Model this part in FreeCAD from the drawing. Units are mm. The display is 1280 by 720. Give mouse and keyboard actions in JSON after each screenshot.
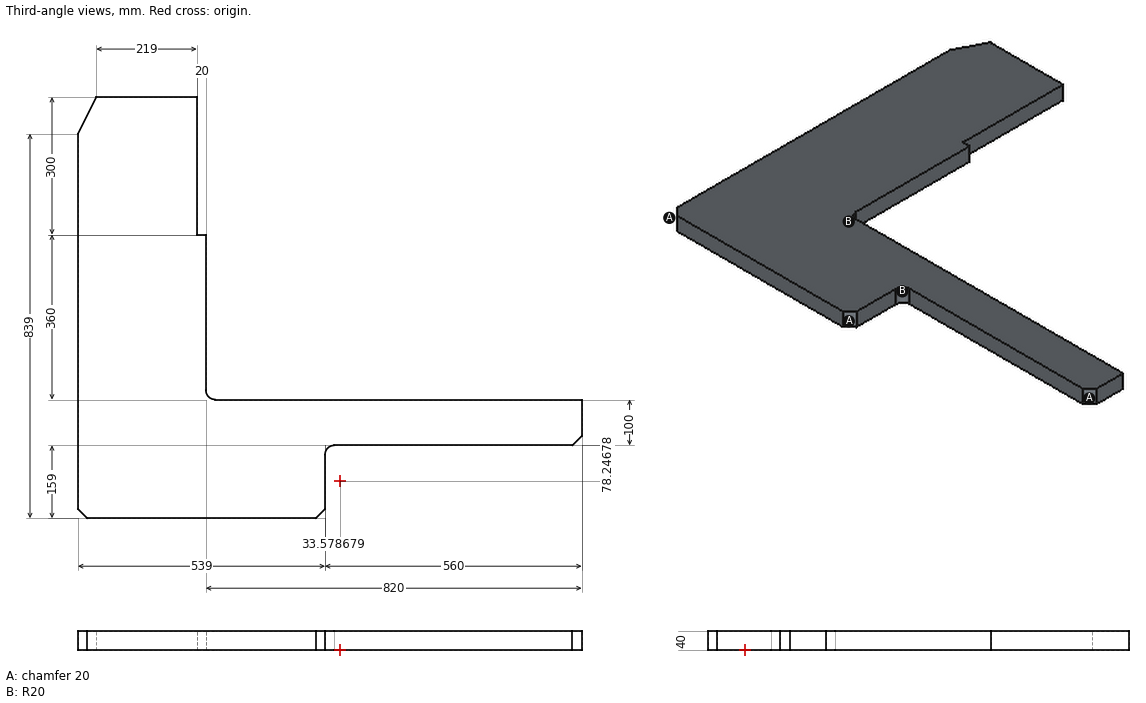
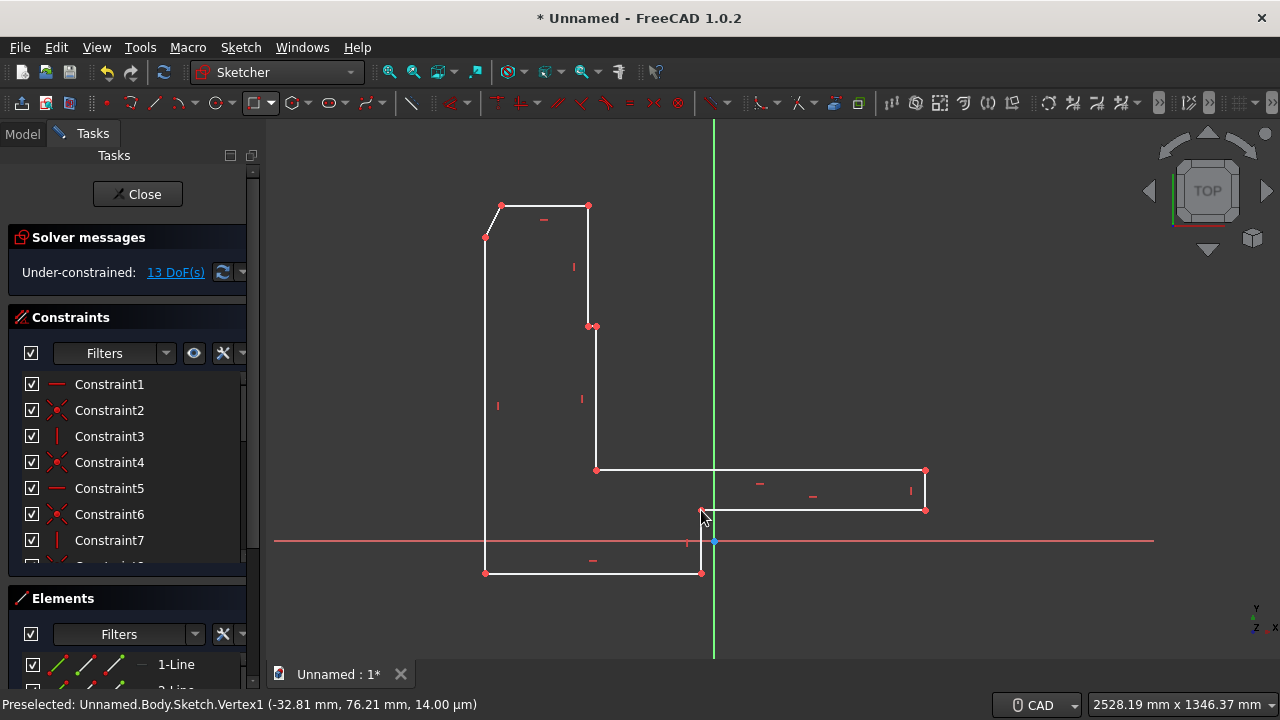
{"action": "scroll", "coordinate": [592, 326], "scroll_direction": "up", "scroll_amount": 7}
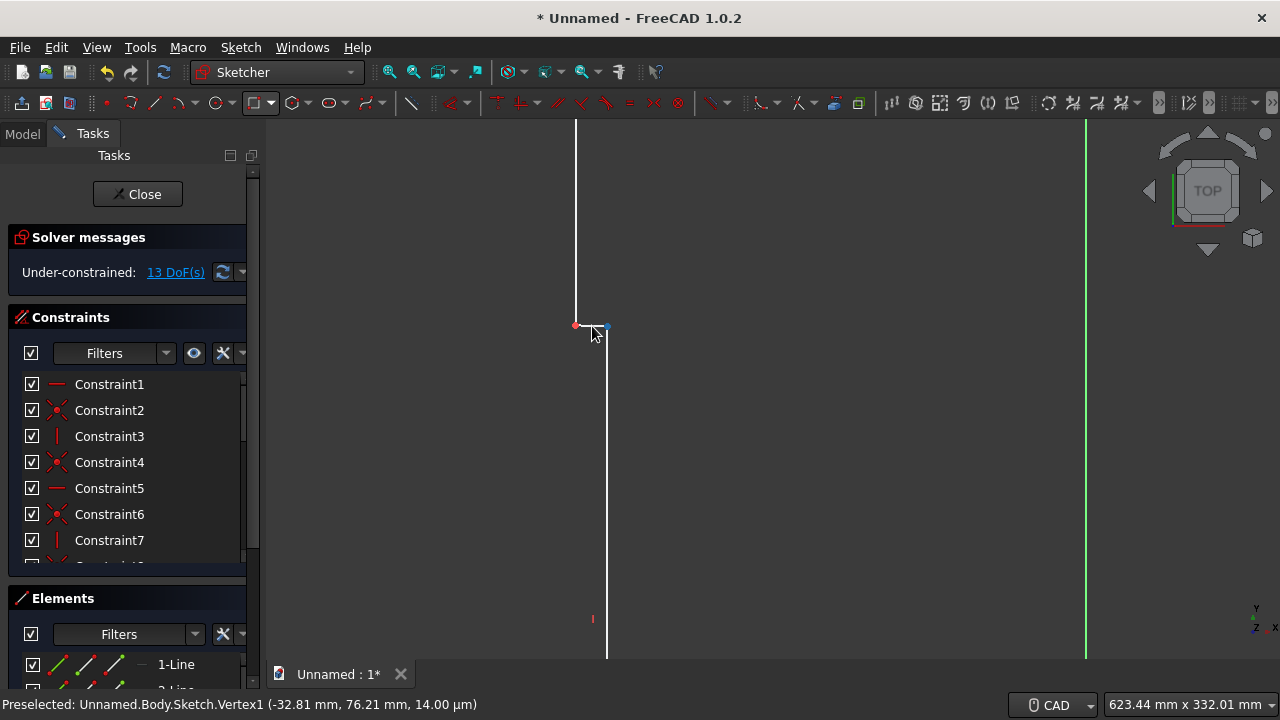
{"action": "left_click", "coordinate": [591, 326]}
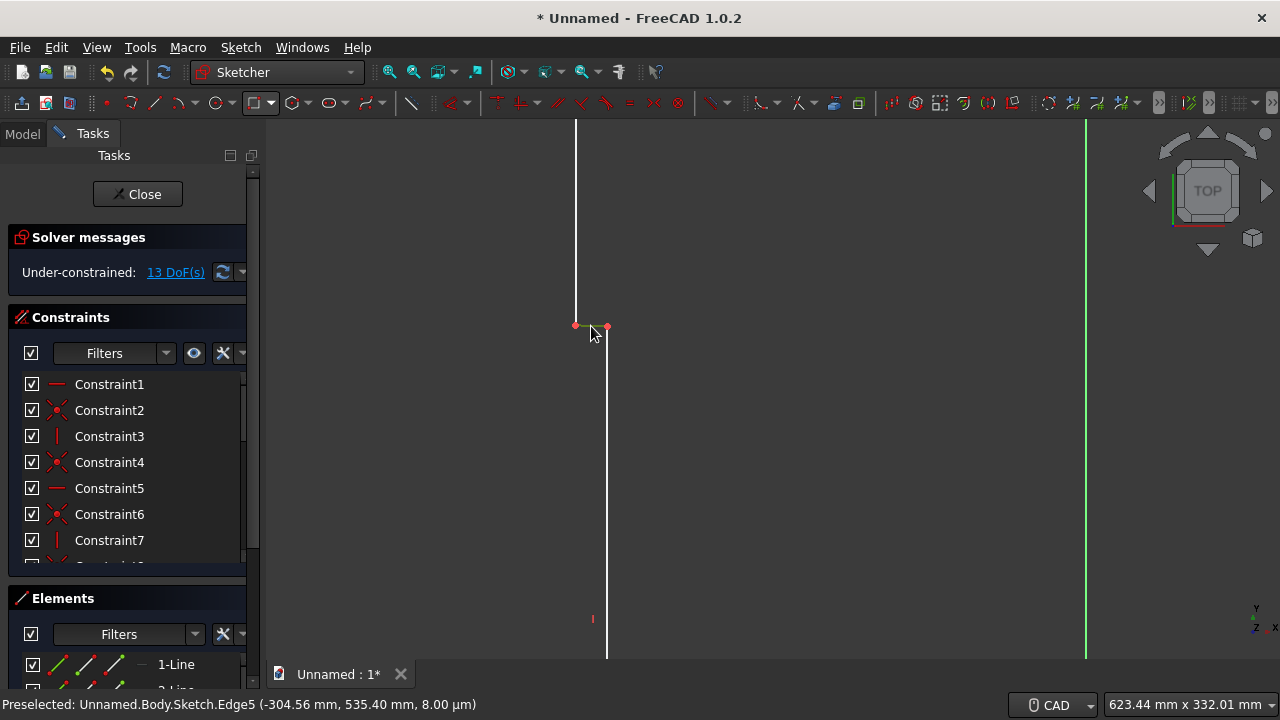
{"action": "key", "text": "h"}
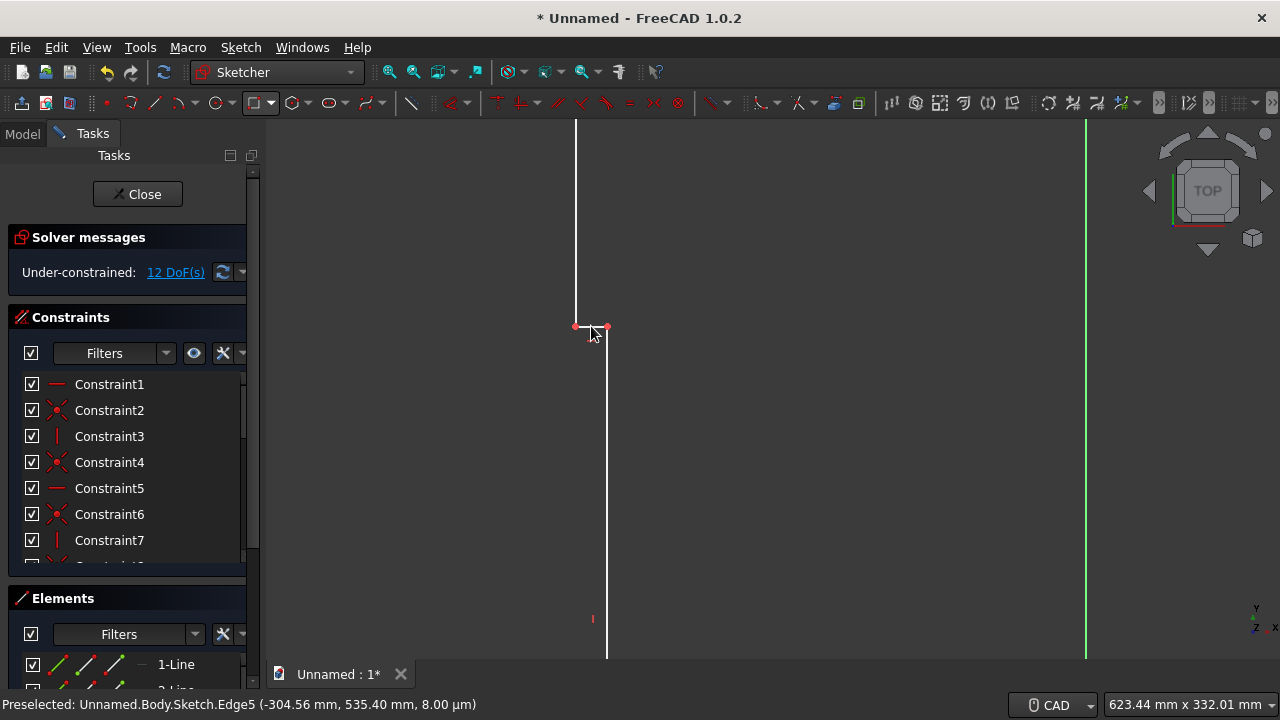
{"action": "key", "text": "d"}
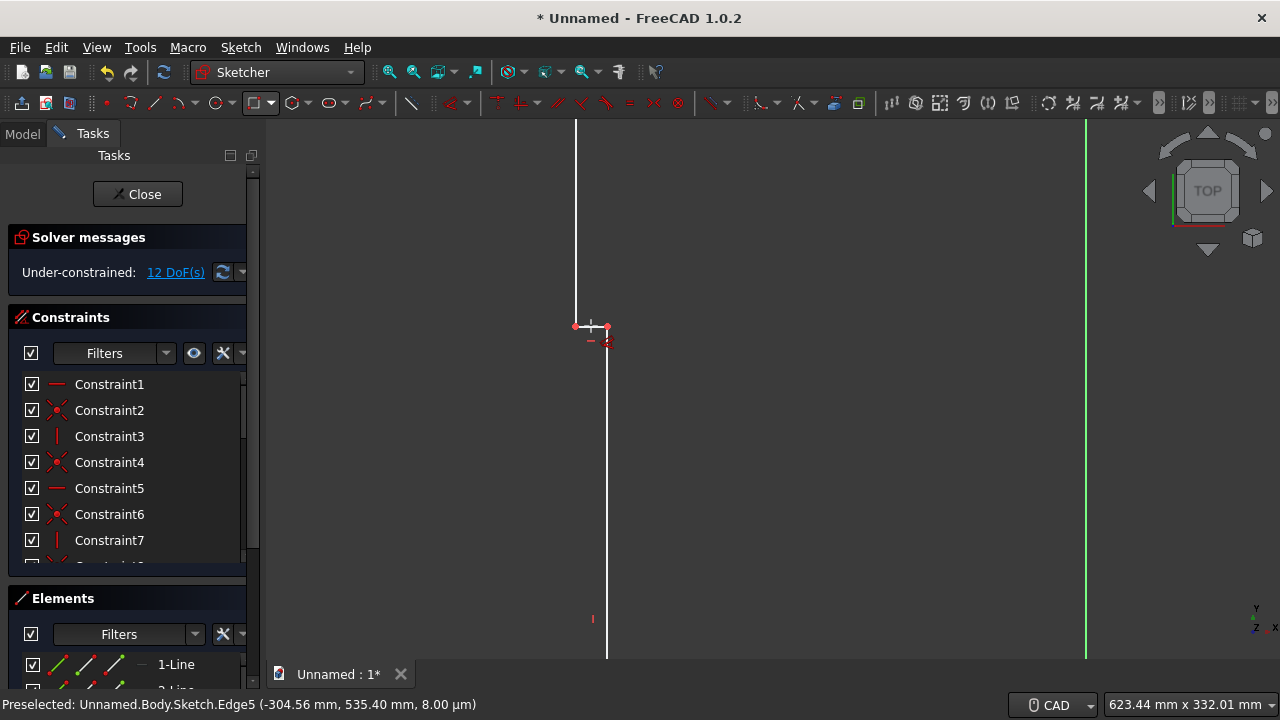
{"action": "scroll", "coordinate": [598, 327], "scroll_direction": "up", "scroll_amount": 2}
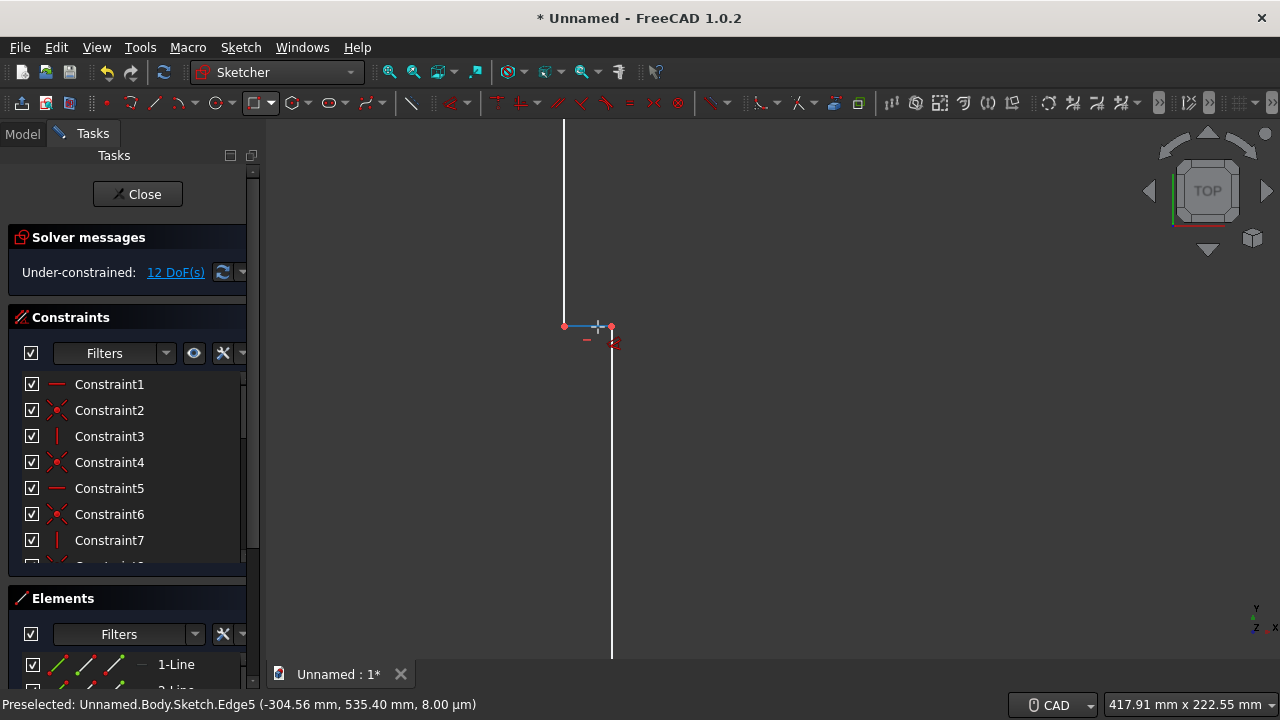
{"action": "left_click", "coordinate": [597, 326]}
{"action": "left_click", "coordinate": [588, 292]}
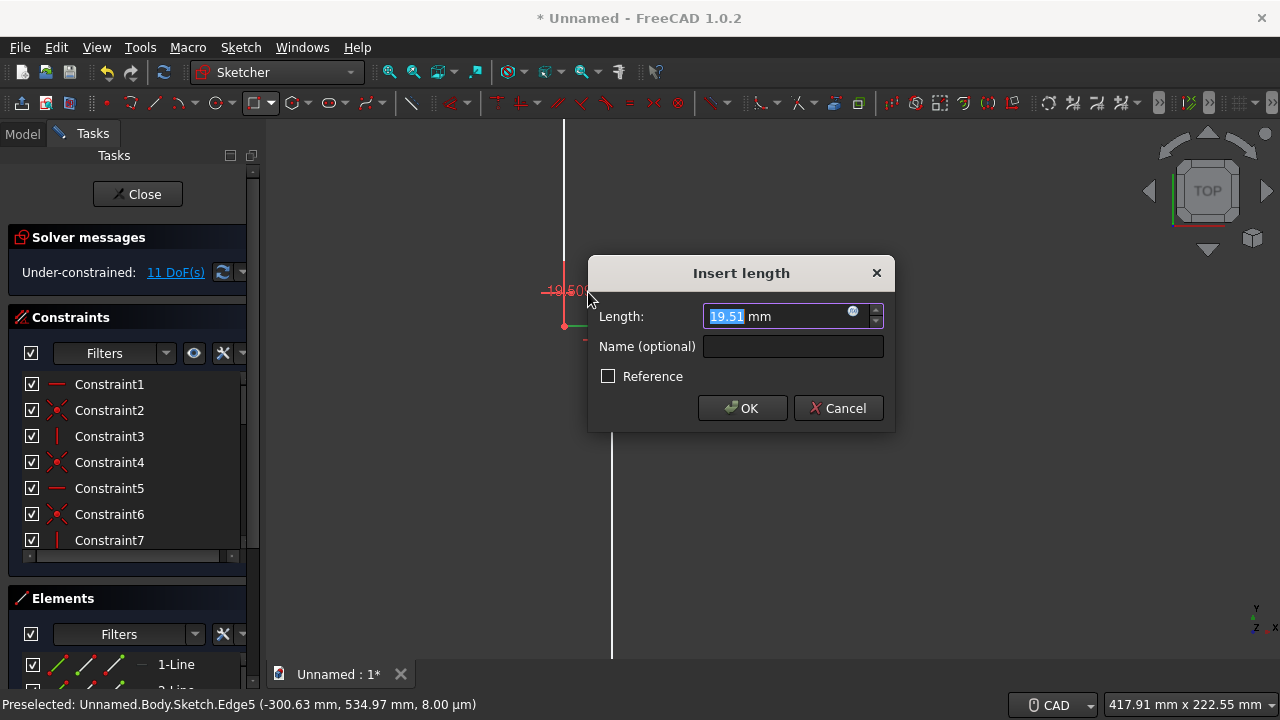
{"action": "type", "text": "20"}
{"action": "key", "text": "Return"}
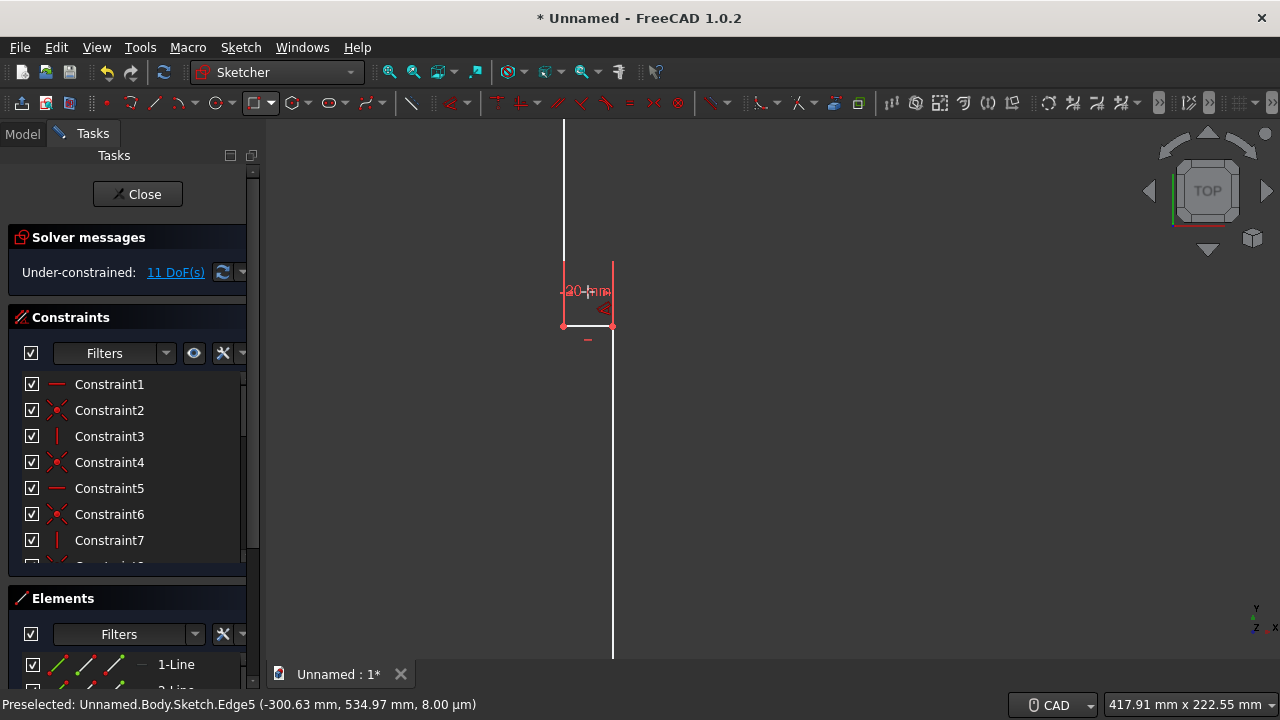
{"action": "scroll", "coordinate": [592, 326], "scroll_direction": "down", "scroll_amount": 9}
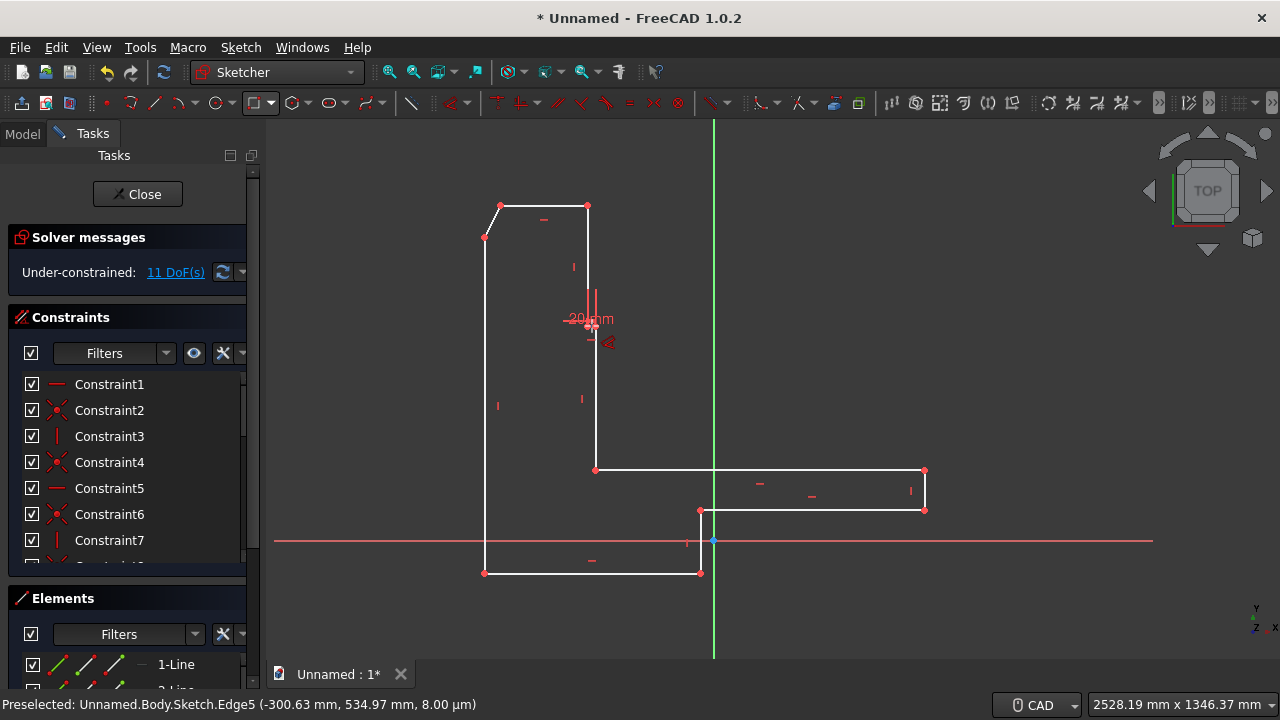
{"action": "left_click", "coordinate": [768, 510]}
{"action": "left_click", "coordinate": [813, 568]}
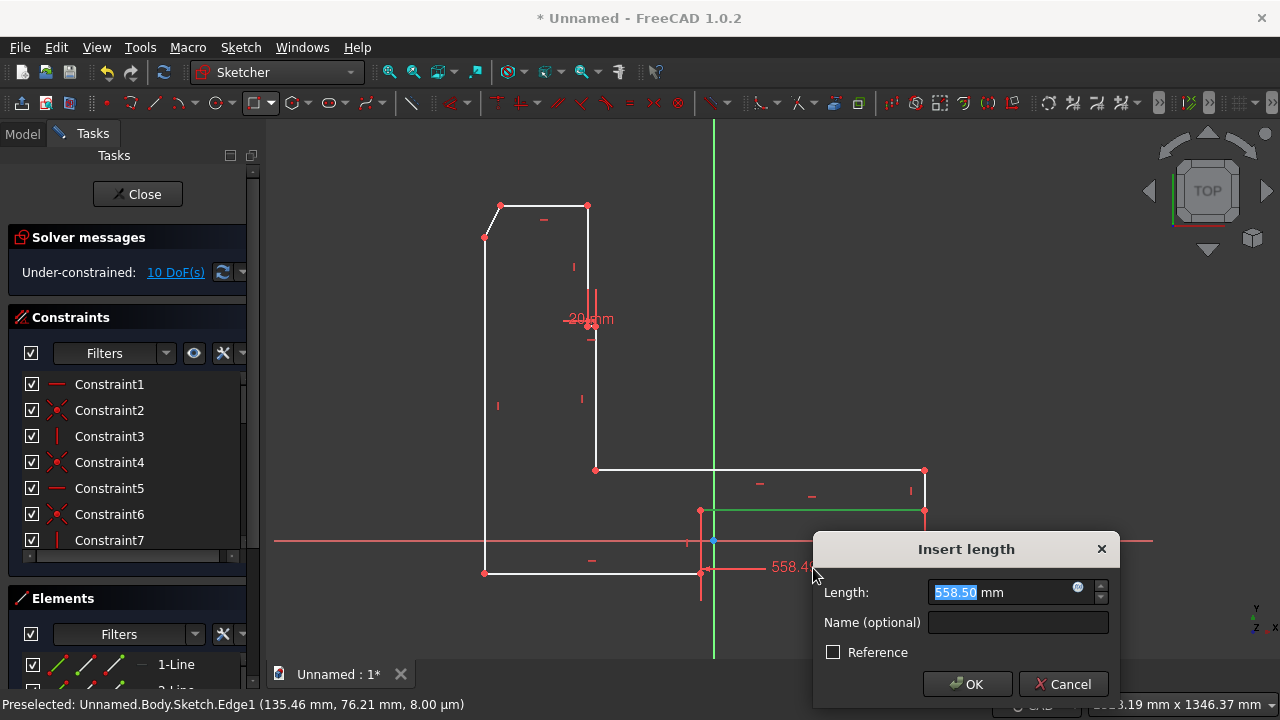
{"action": "type", "text": "560"}
{"action": "key", "text": "Return"}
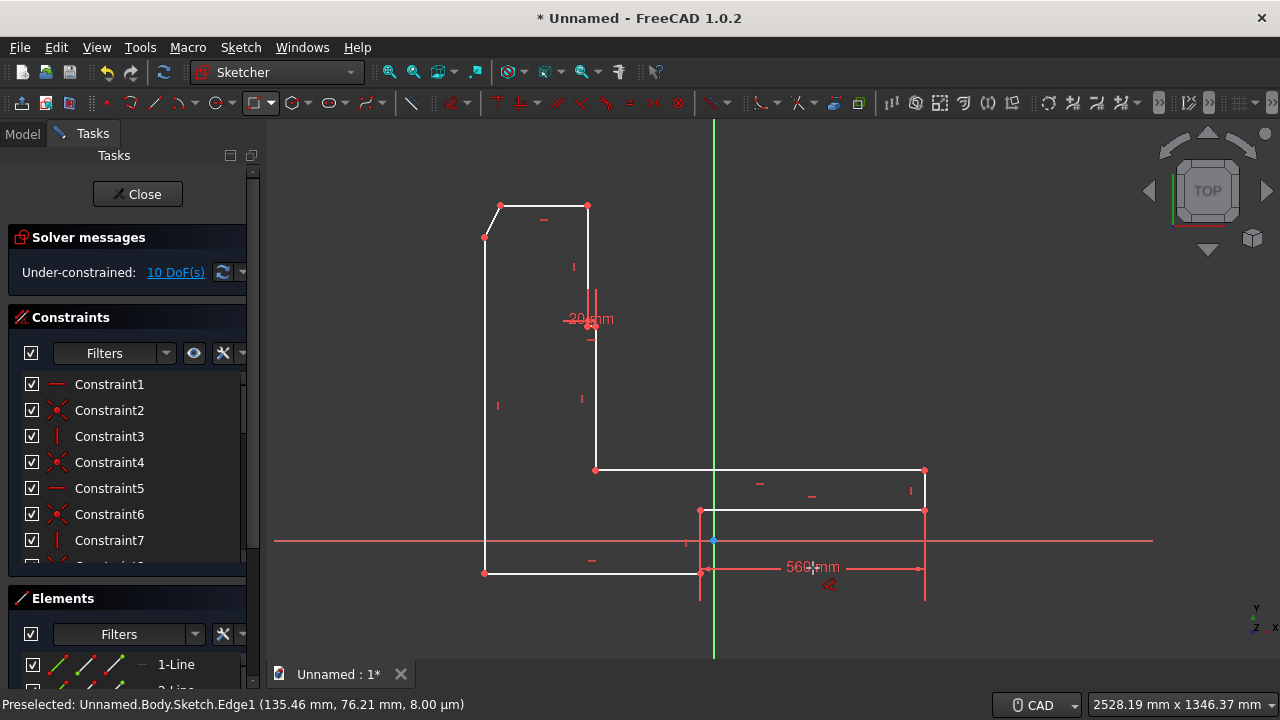
{"action": "left_click", "coordinate": [925, 498]}
{"action": "left_click", "coordinate": [959, 490]}